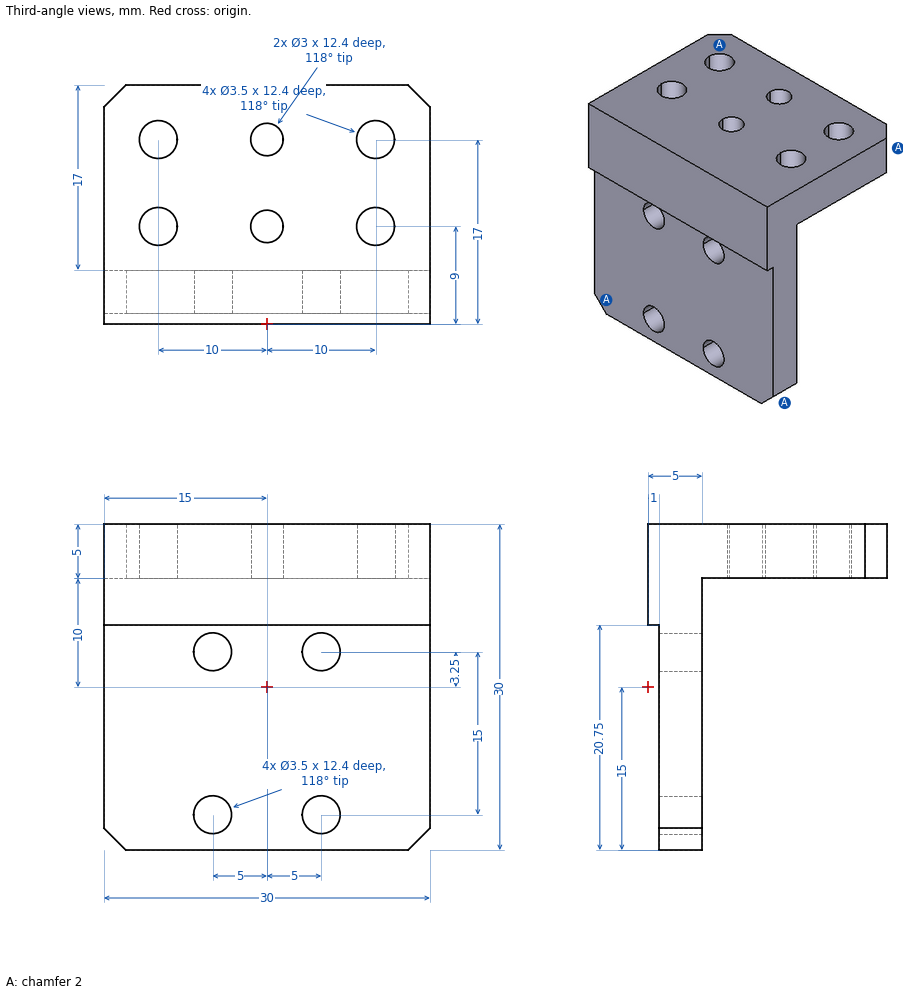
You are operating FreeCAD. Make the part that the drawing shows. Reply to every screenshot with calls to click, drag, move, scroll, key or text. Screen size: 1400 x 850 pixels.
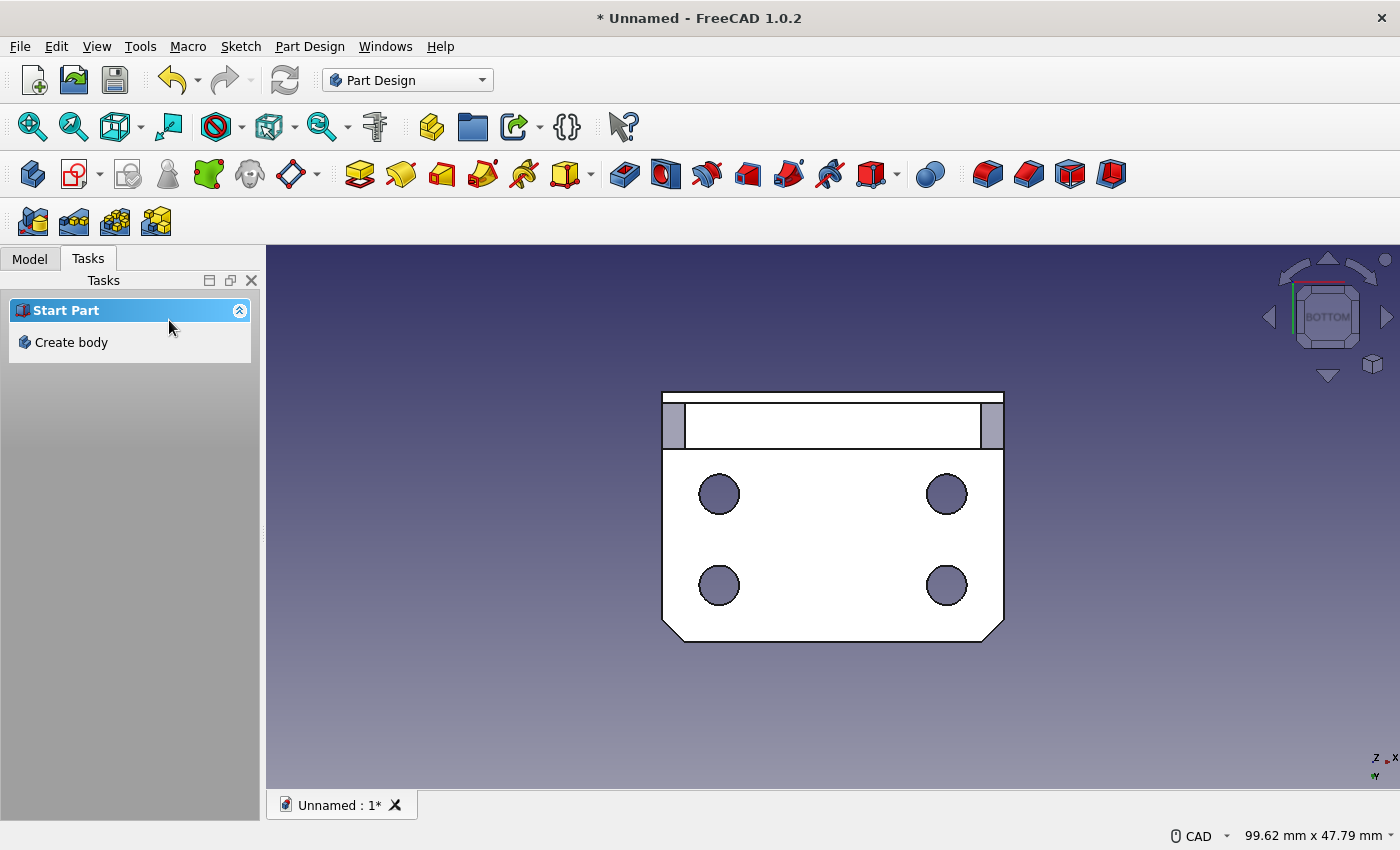
click(833, 544)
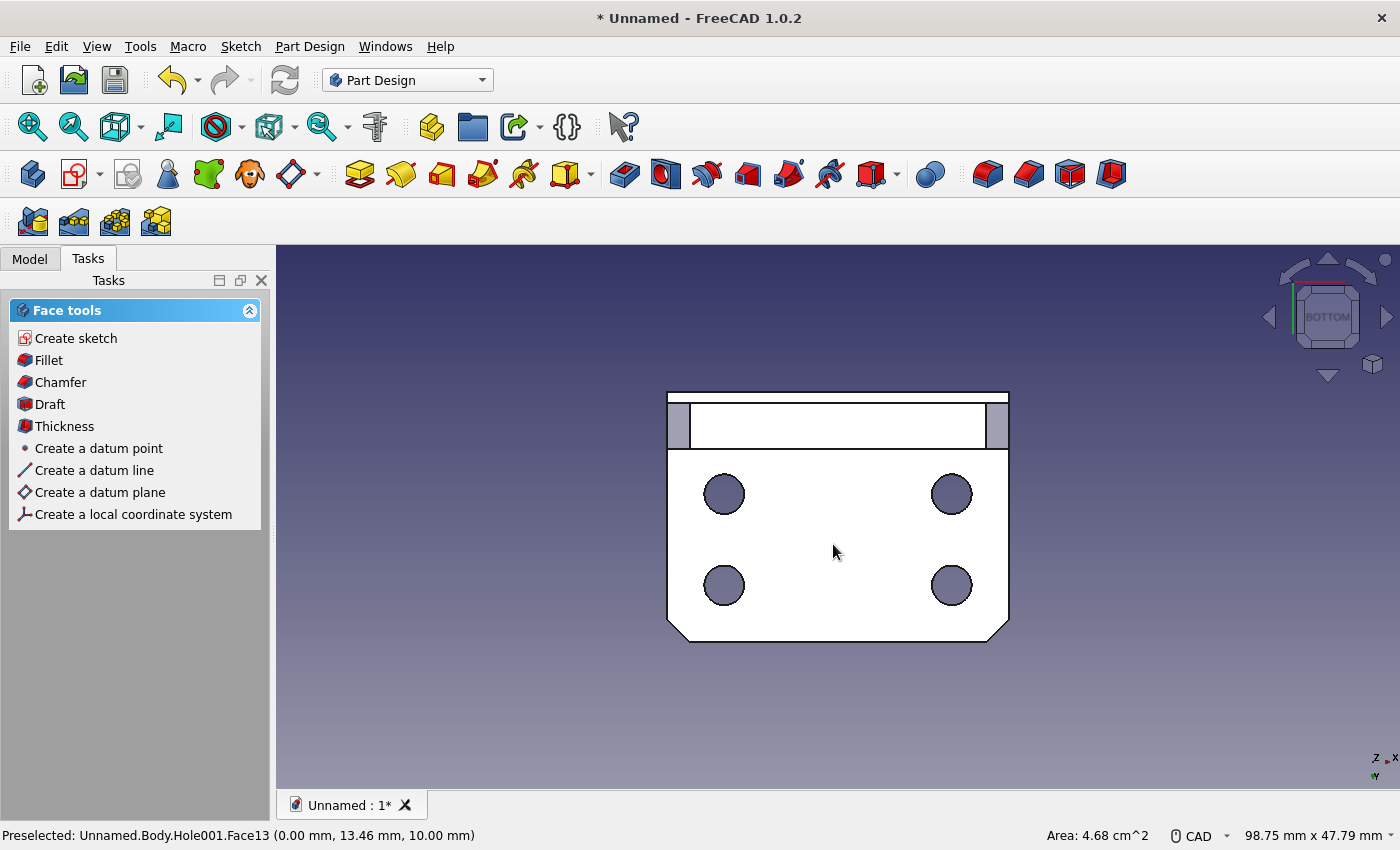
click(74, 174)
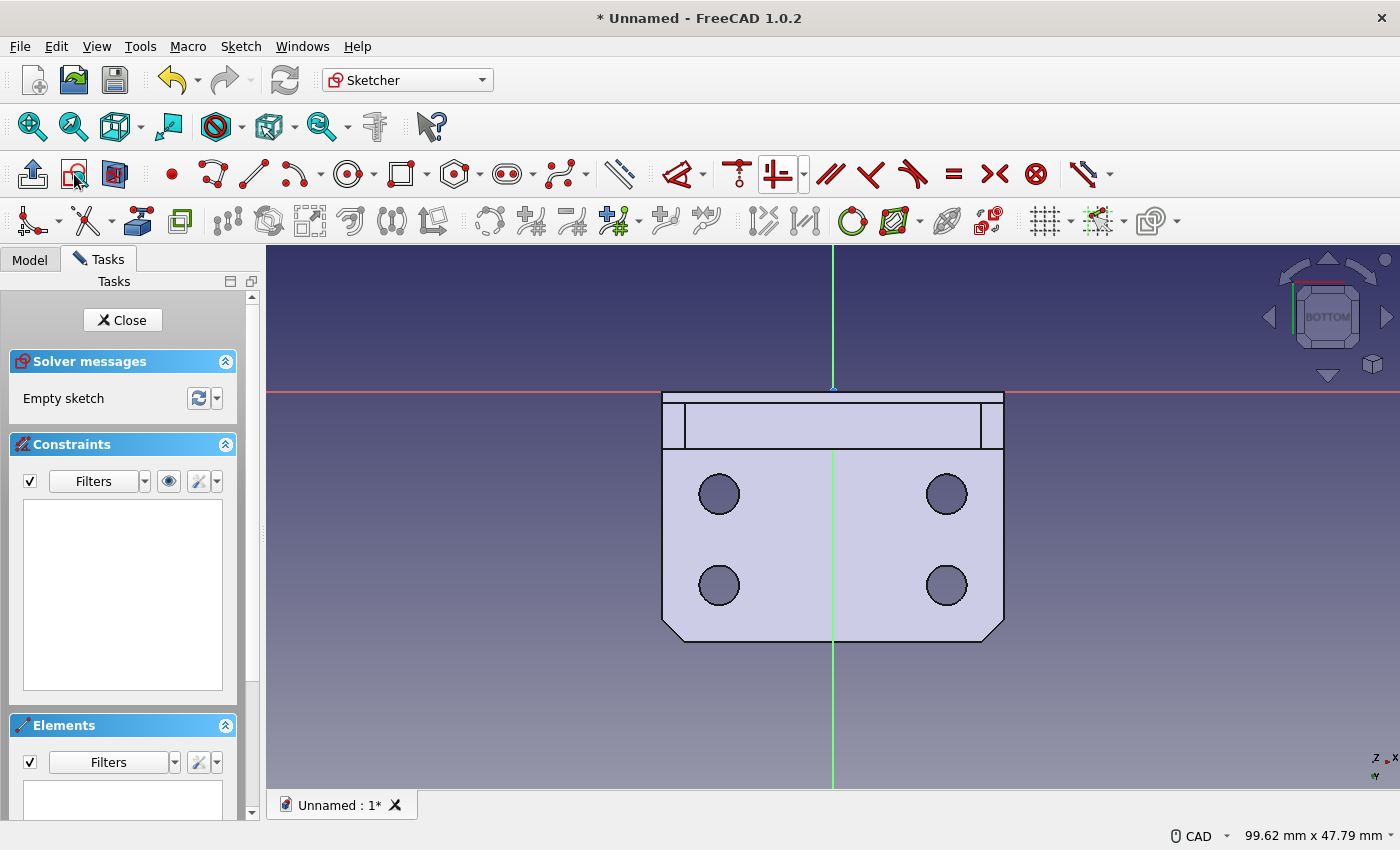
key(q)
key(s)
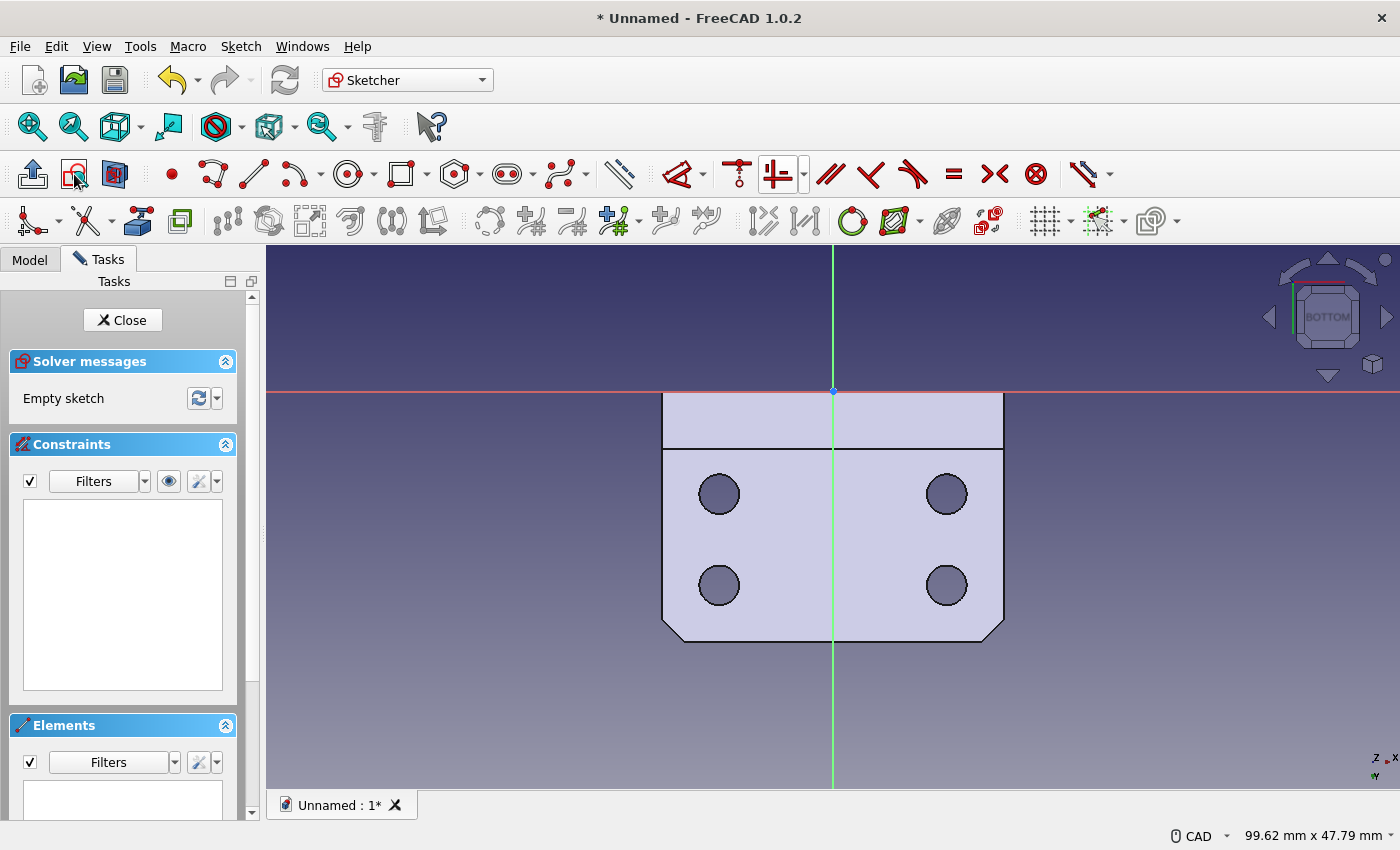
scroll(972, 457, up, 2)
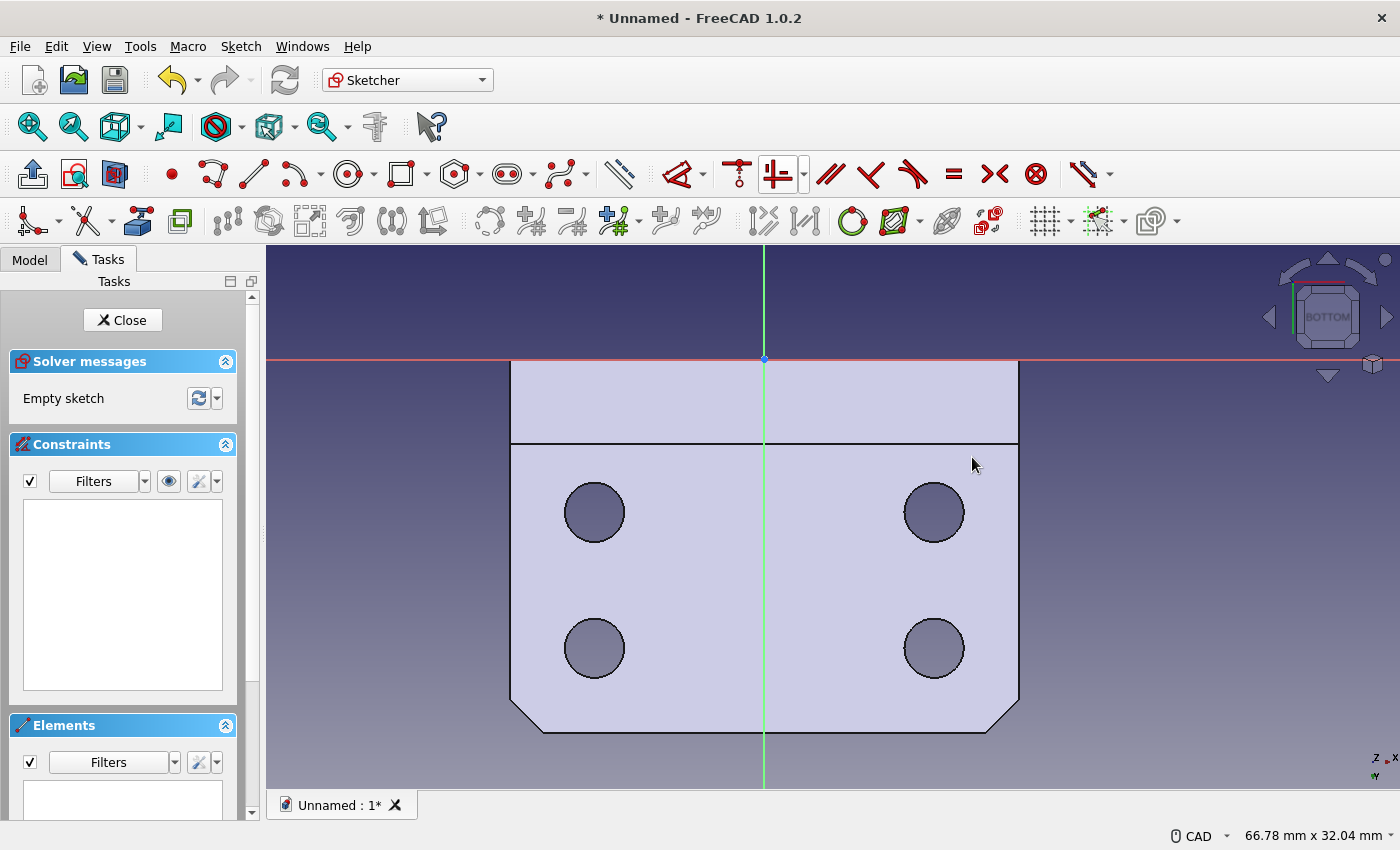
click(348, 174)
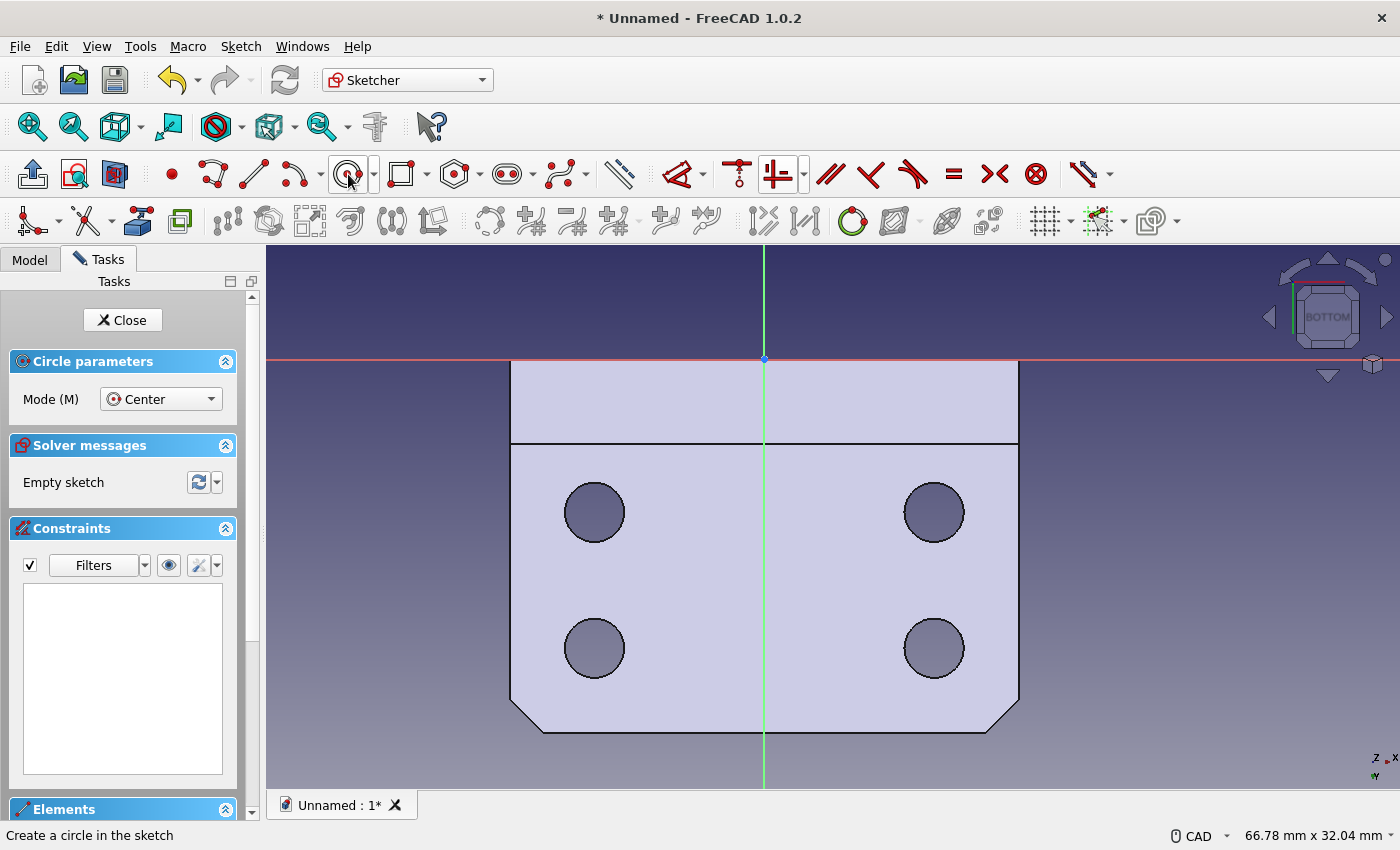
click(764, 648)
click(782, 630)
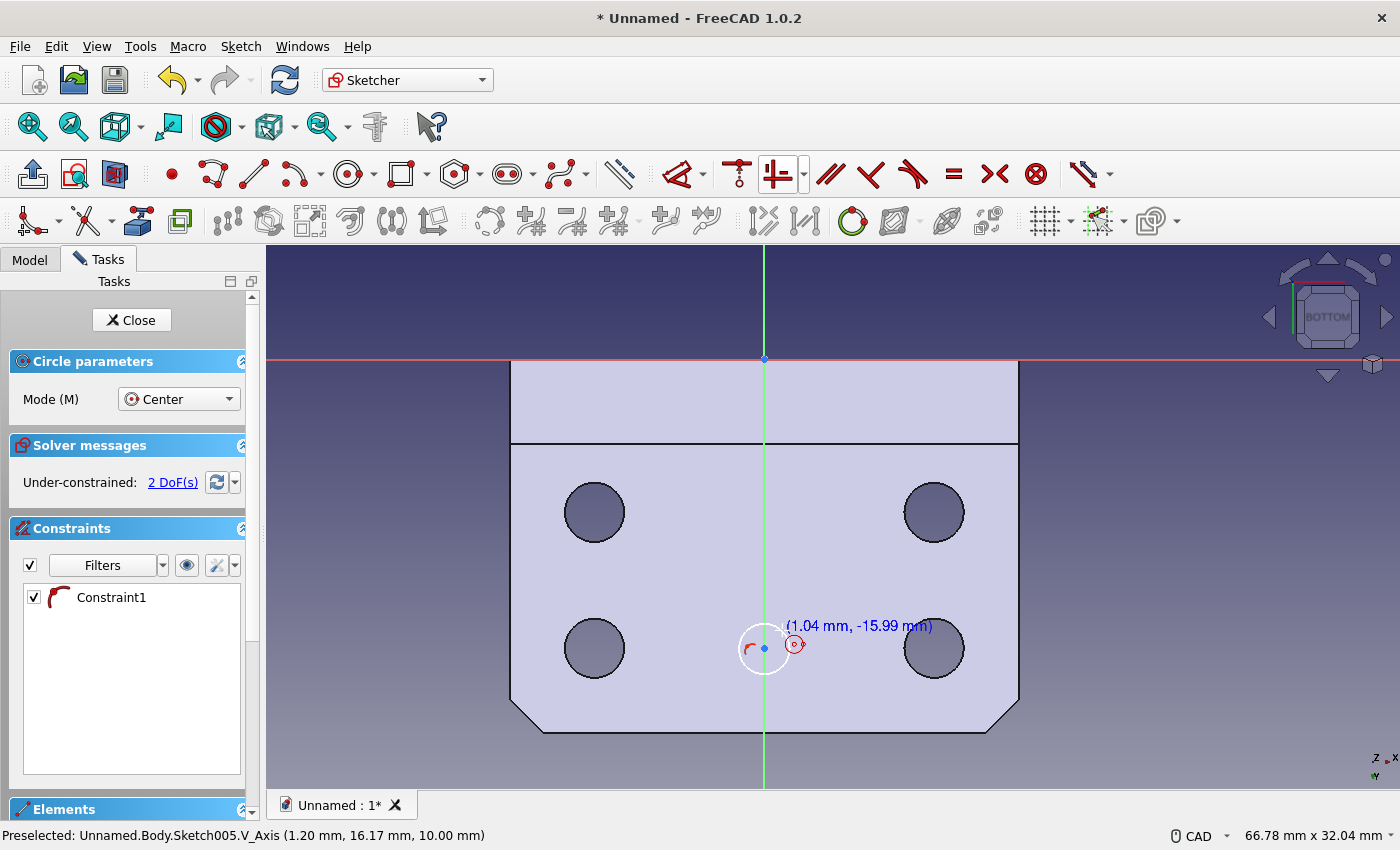
click(764, 512)
click(782, 494)
key(Escape)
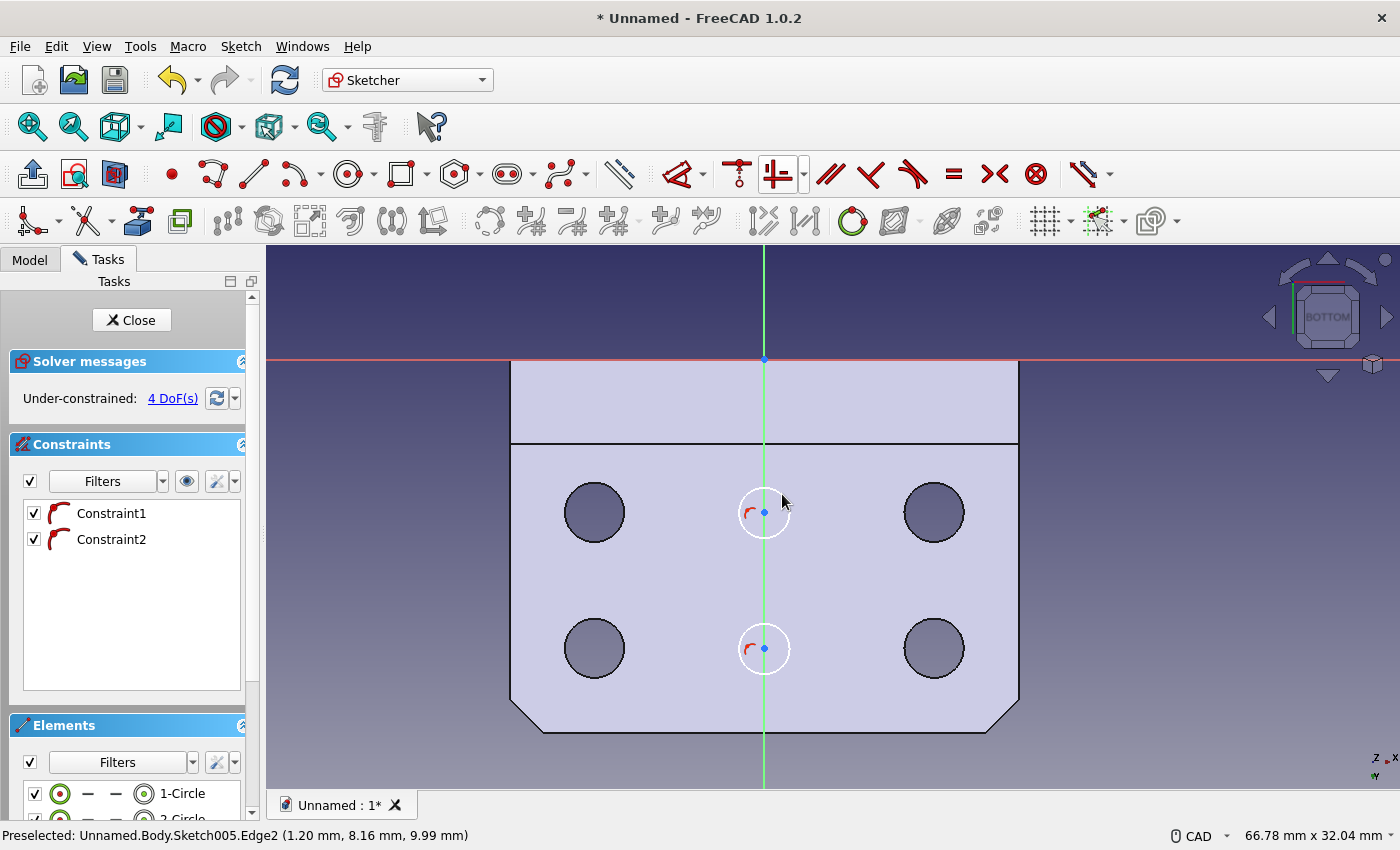
click(782, 631)